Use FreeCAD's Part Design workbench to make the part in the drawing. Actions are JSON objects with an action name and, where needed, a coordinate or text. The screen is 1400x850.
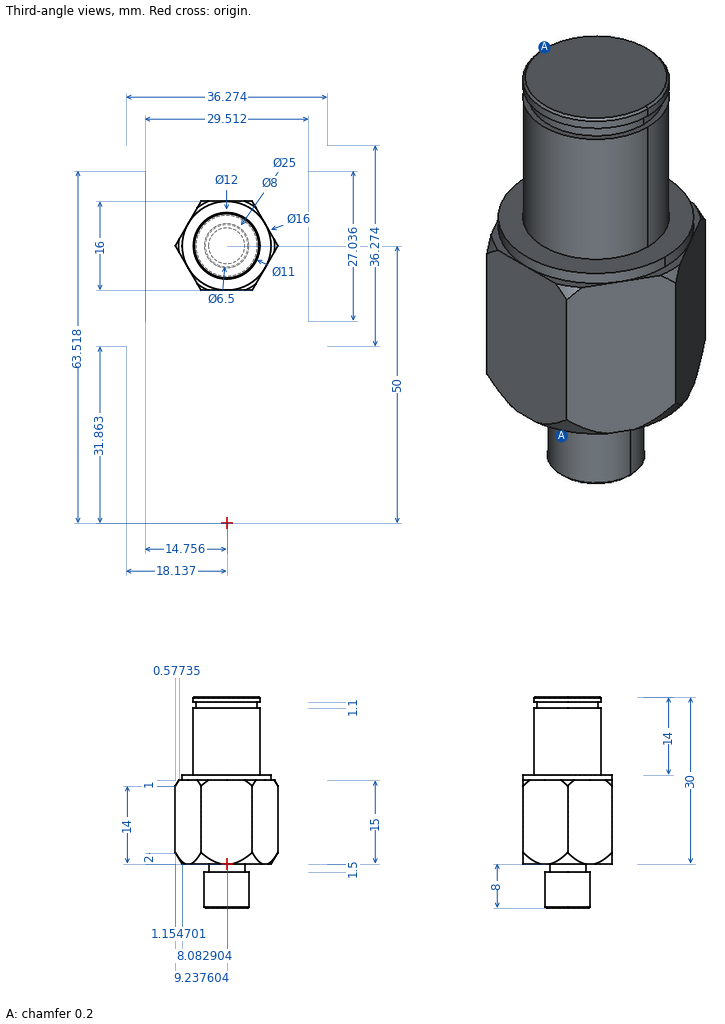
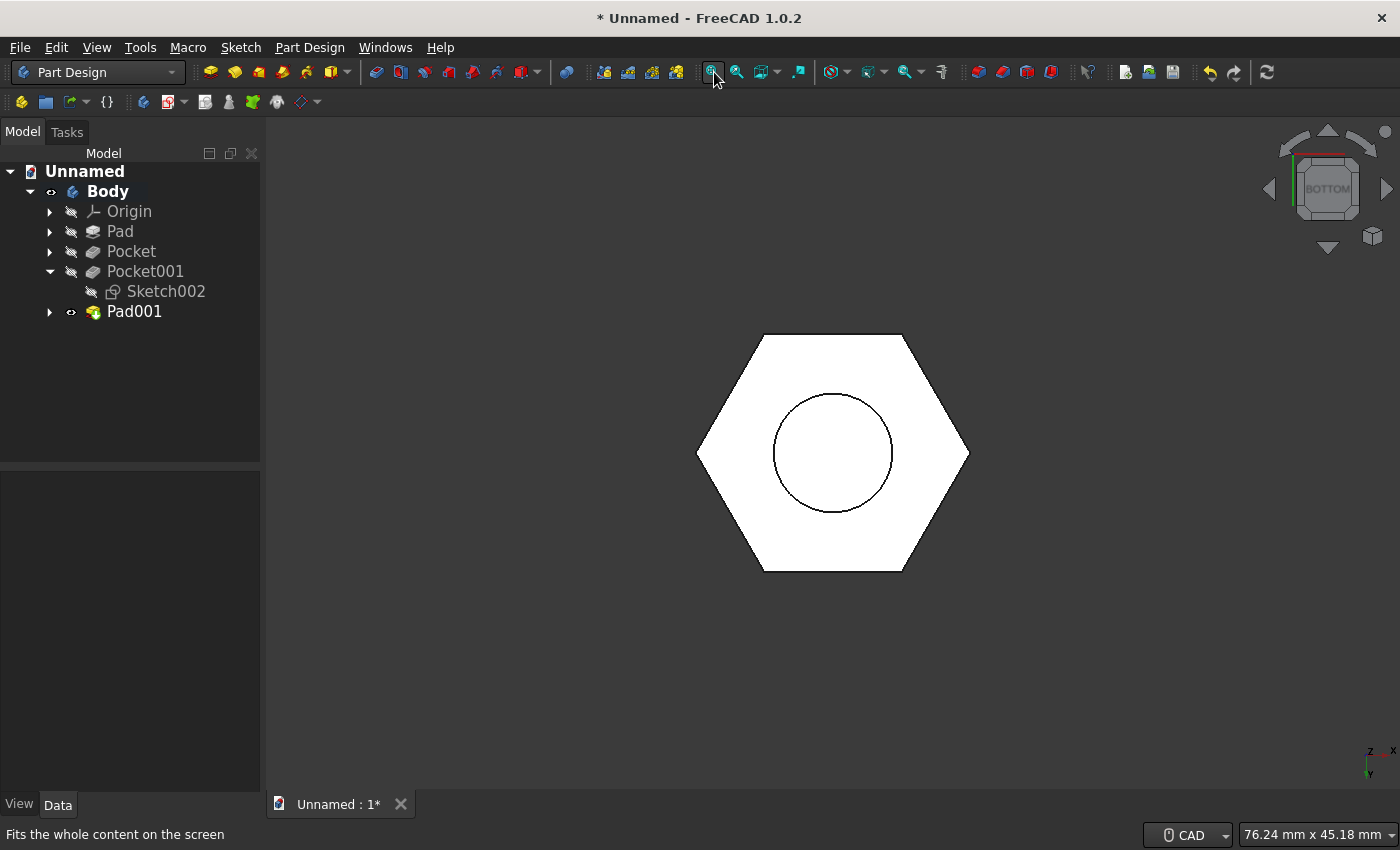
{"action": "left_click", "coordinate": [168, 102]}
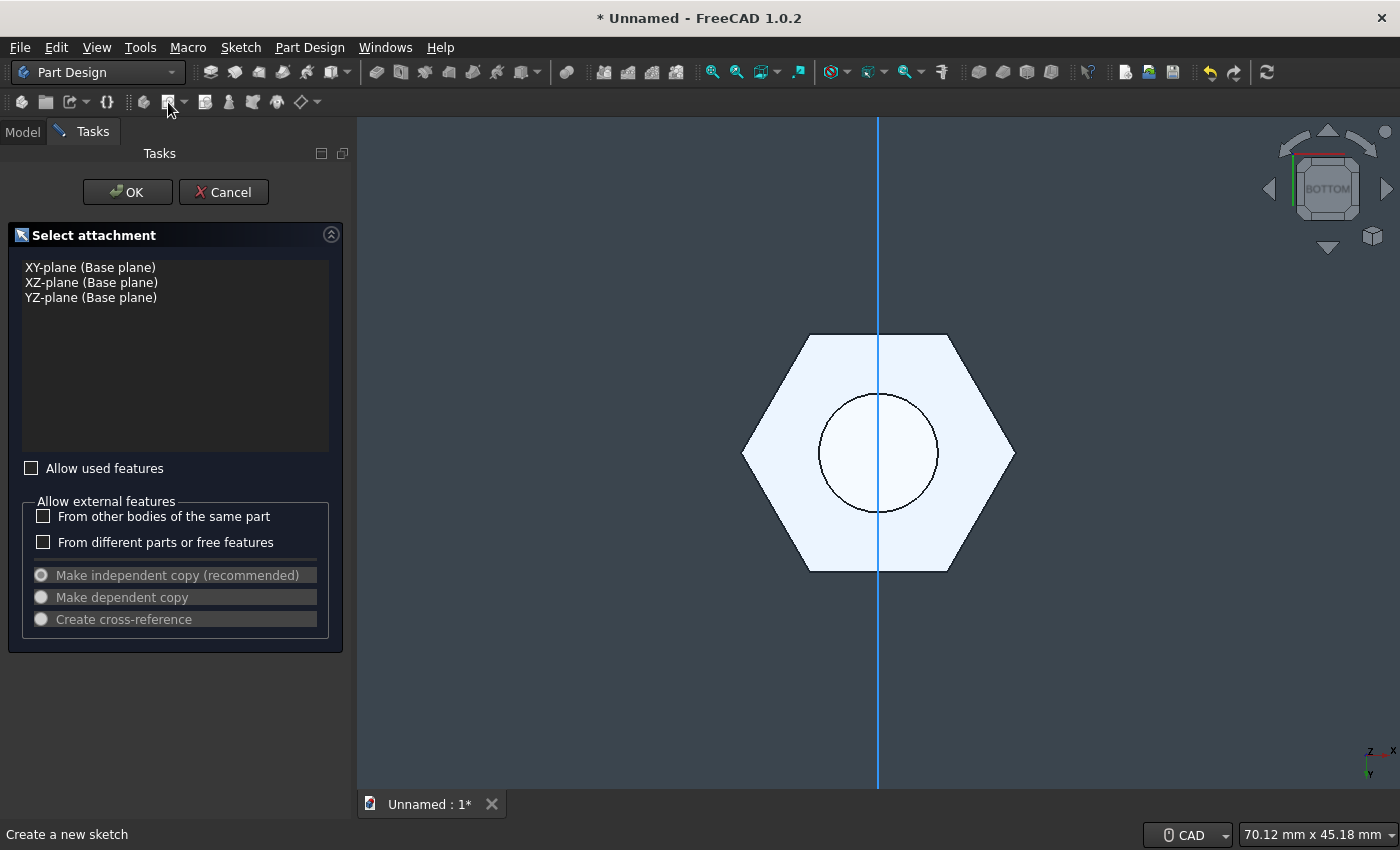
{"action": "left_click", "coordinate": [82, 268]}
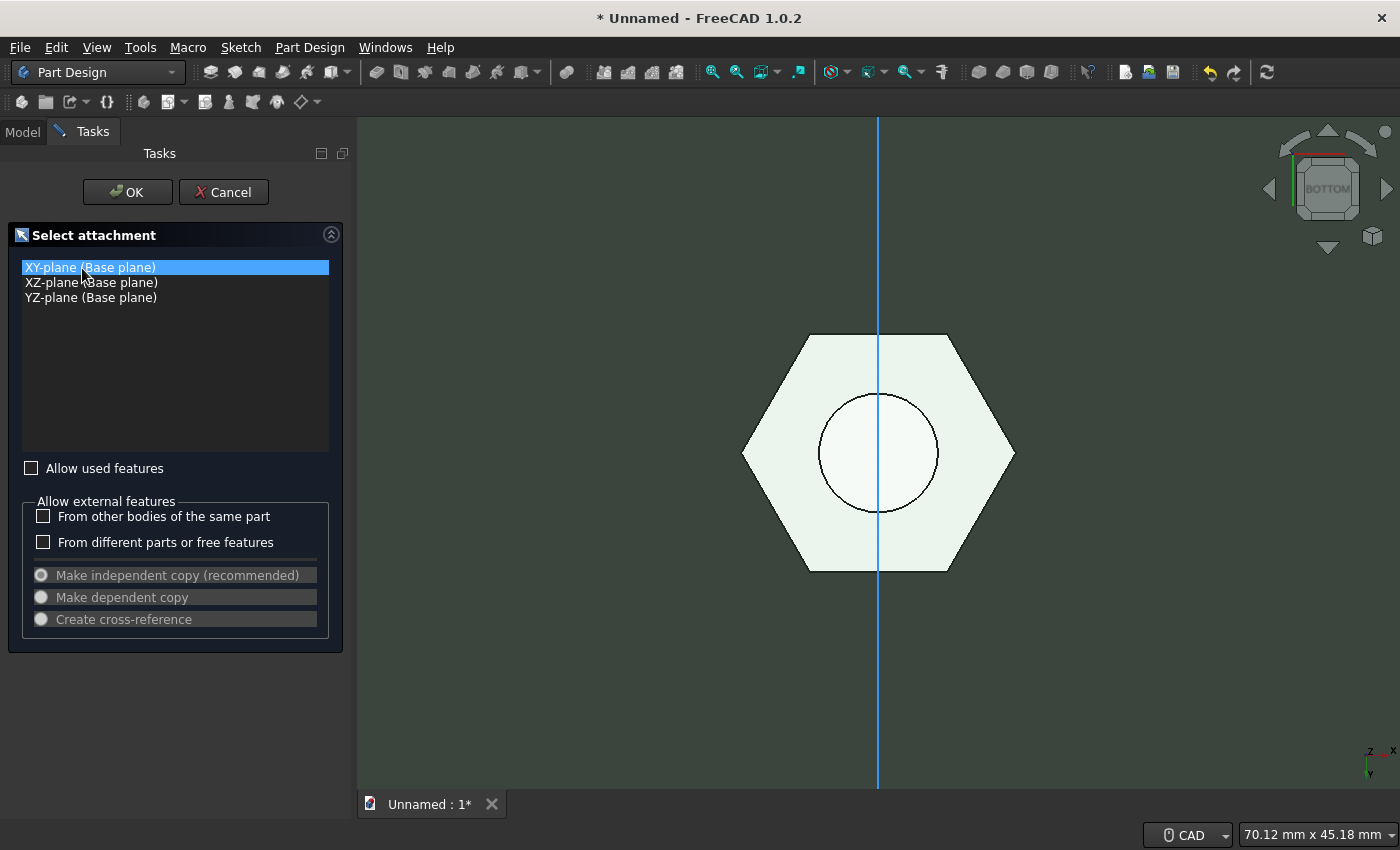
{"action": "left_click", "coordinate": [128, 192]}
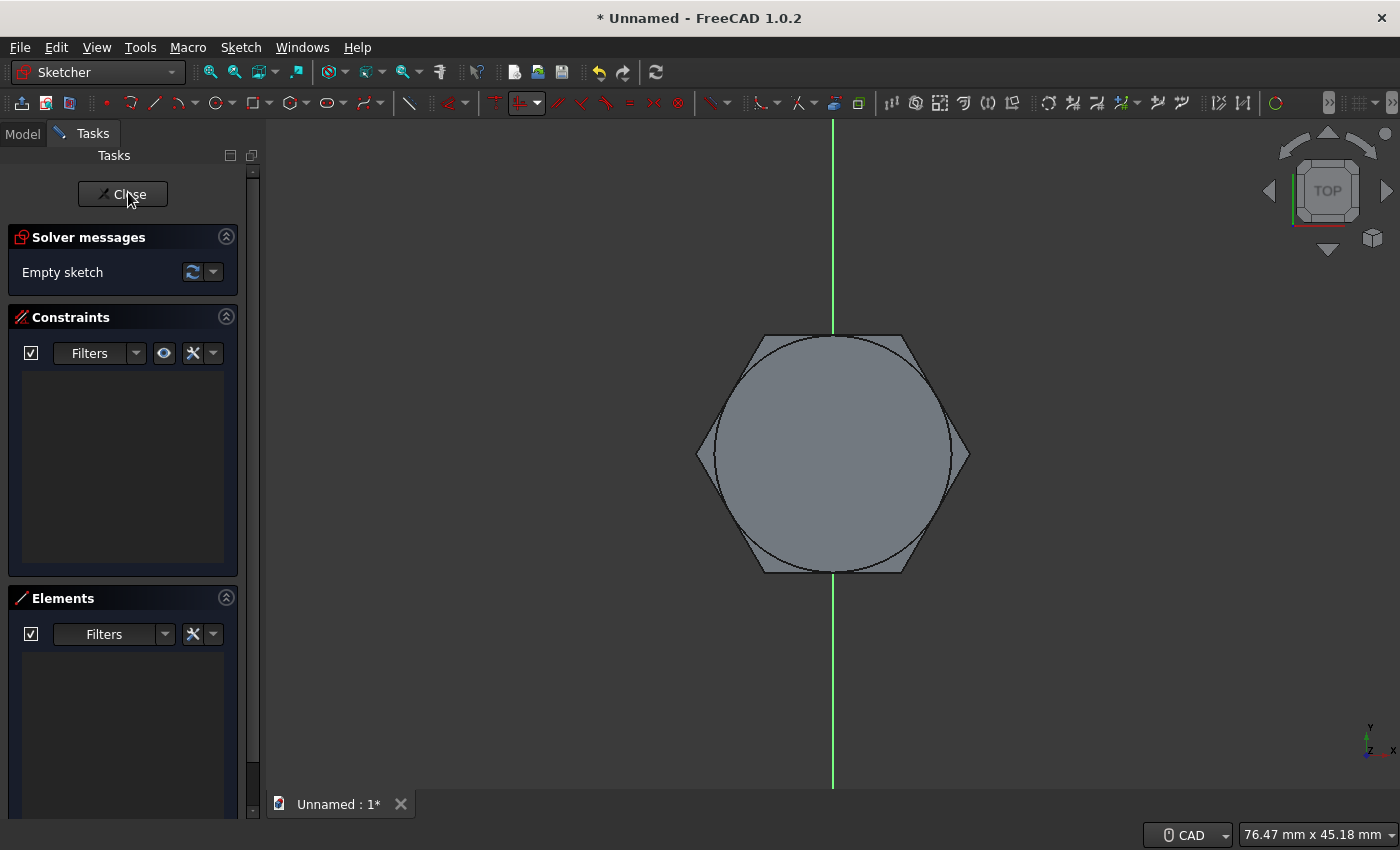
{"action": "left_click", "coordinate": [70, 104]}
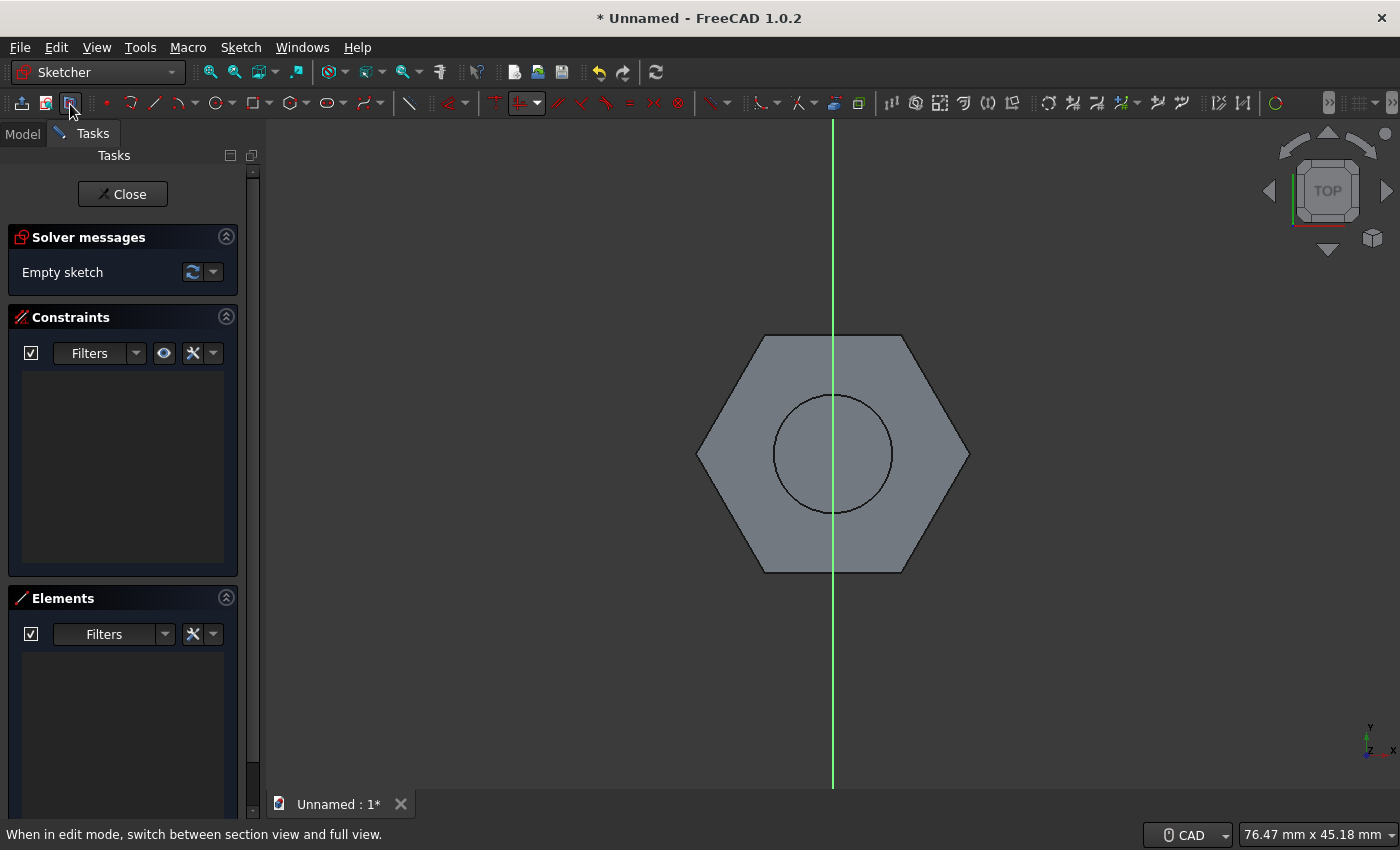
{"action": "scroll", "coordinate": [709, 233], "scroll_direction": "down", "scroll_amount": 4}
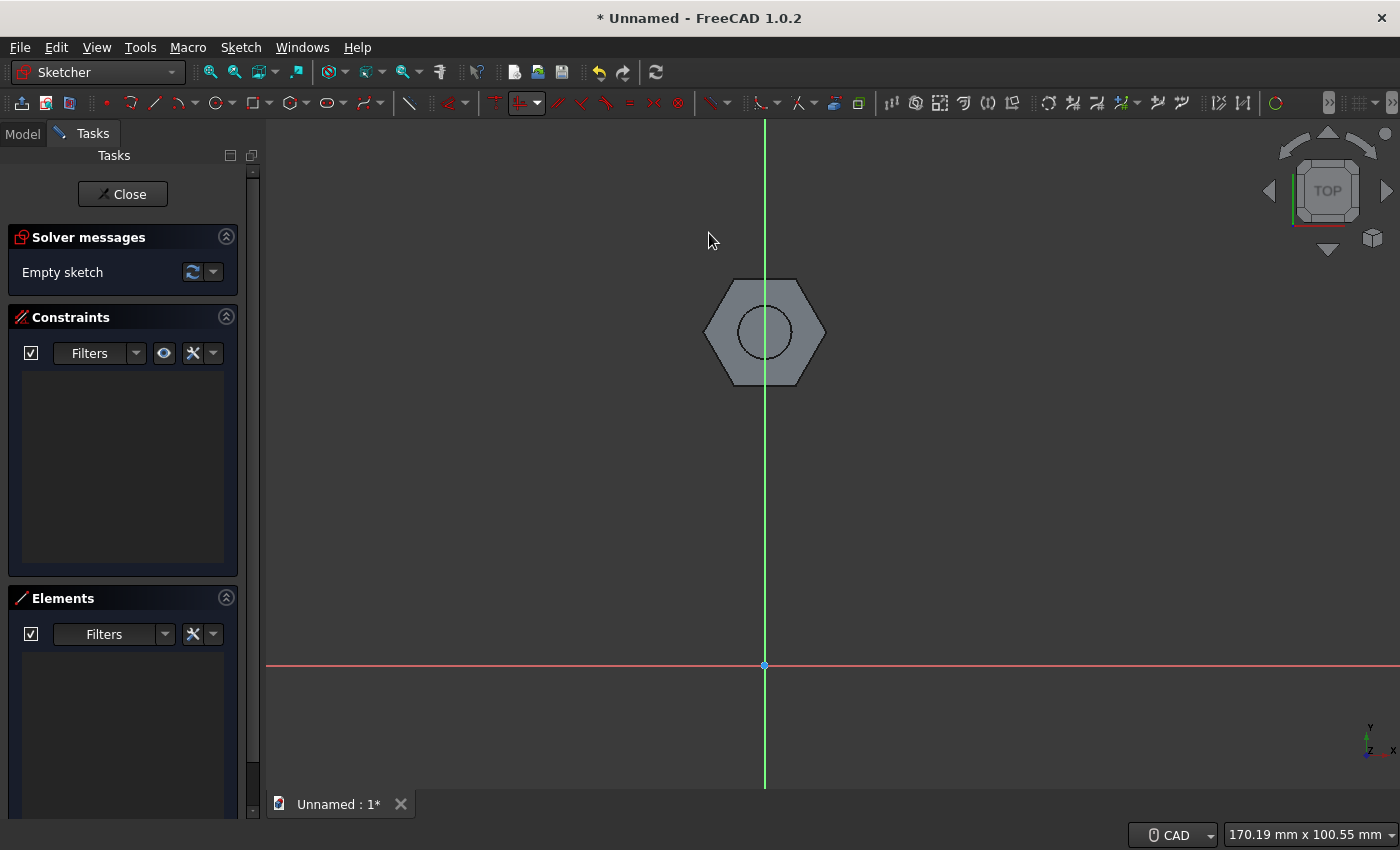
{"action": "left_click", "coordinate": [254, 104]}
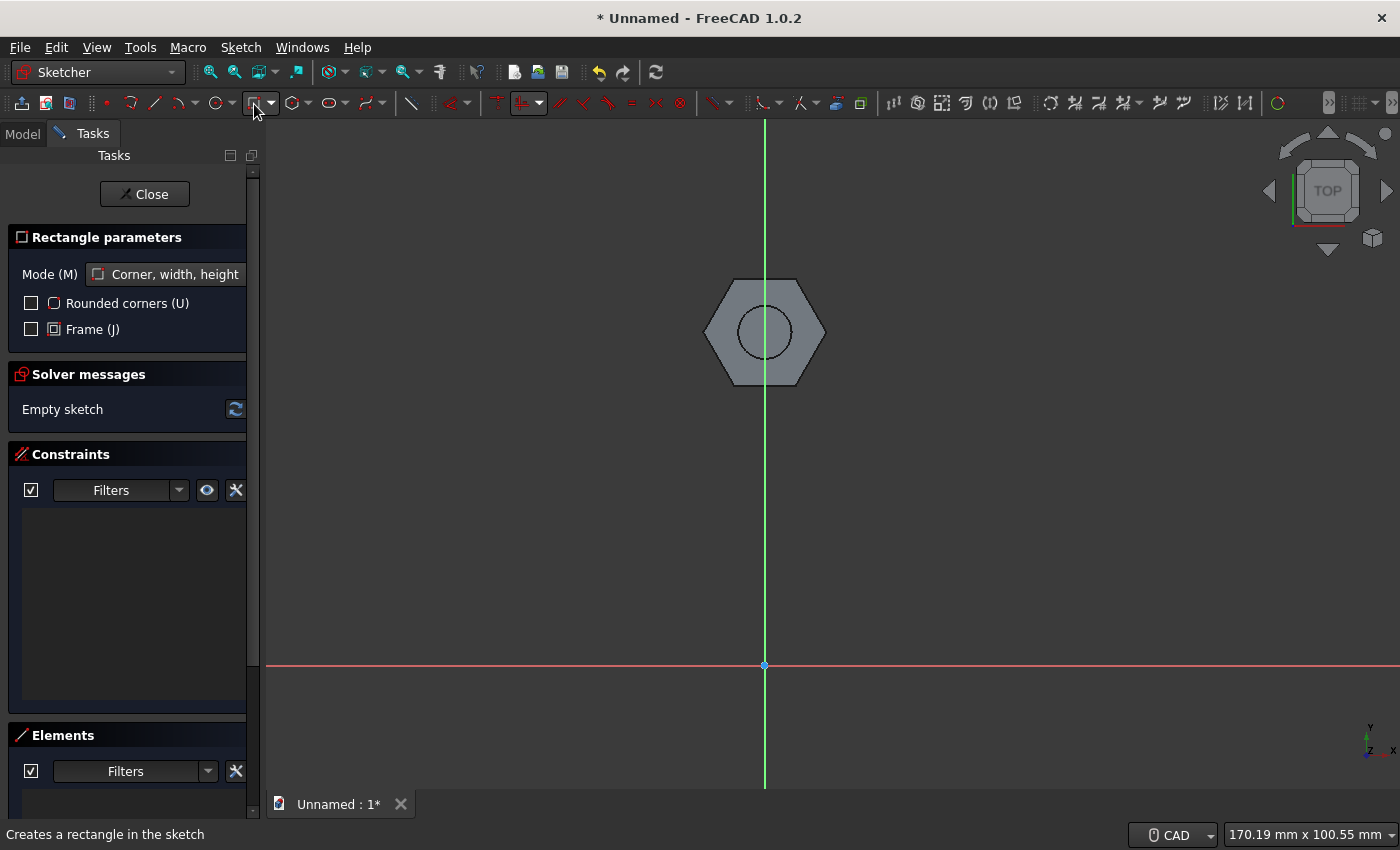
{"action": "left_click", "coordinate": [667, 242]}
{"action": "mouse_move", "coordinate": [863, 422]}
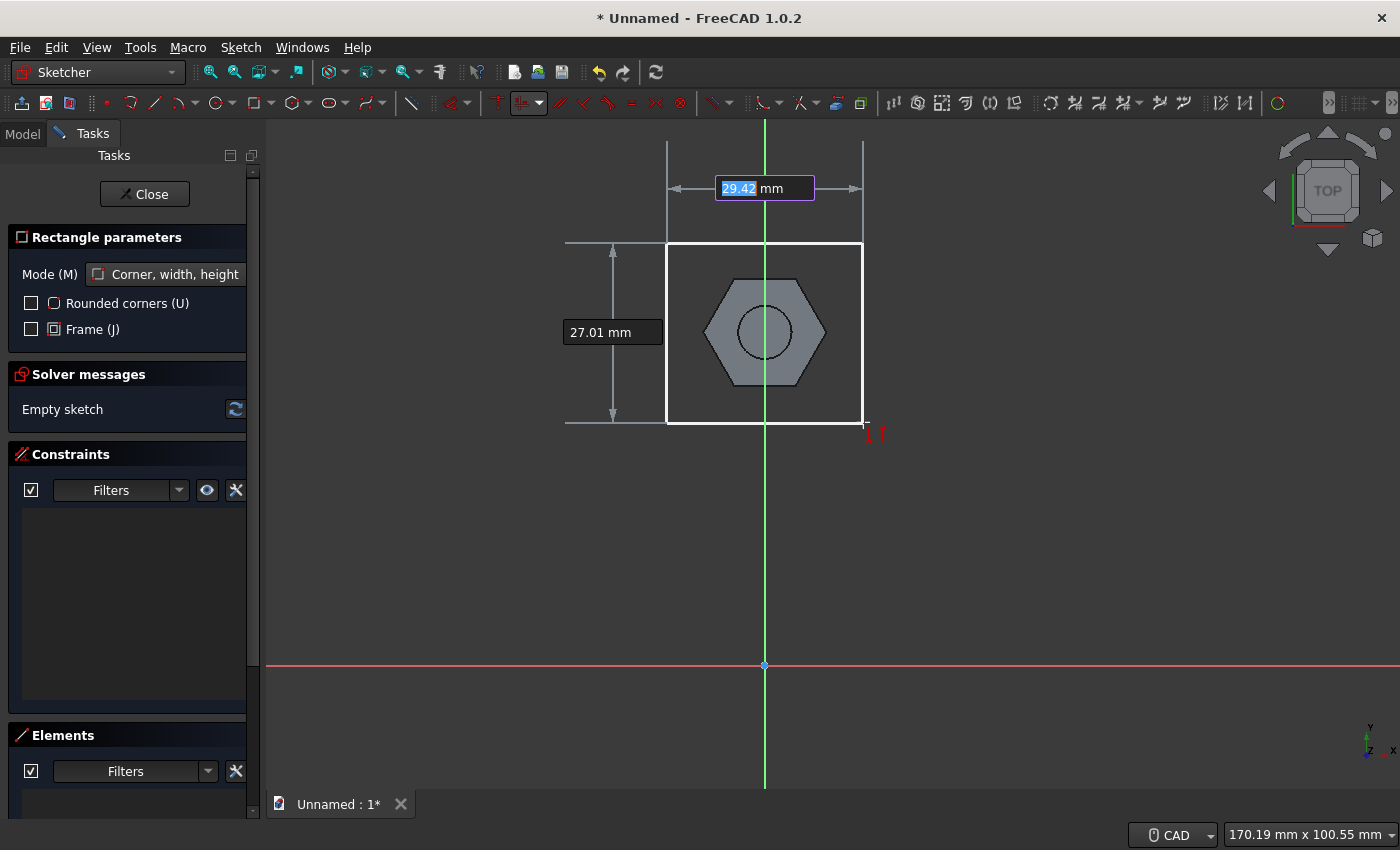
{"action": "type", "text": "29.512"}
{"action": "key", "text": "Tab"}
{"action": "type", "text": "27.036"}
{"action": "key", "text": "Return"}